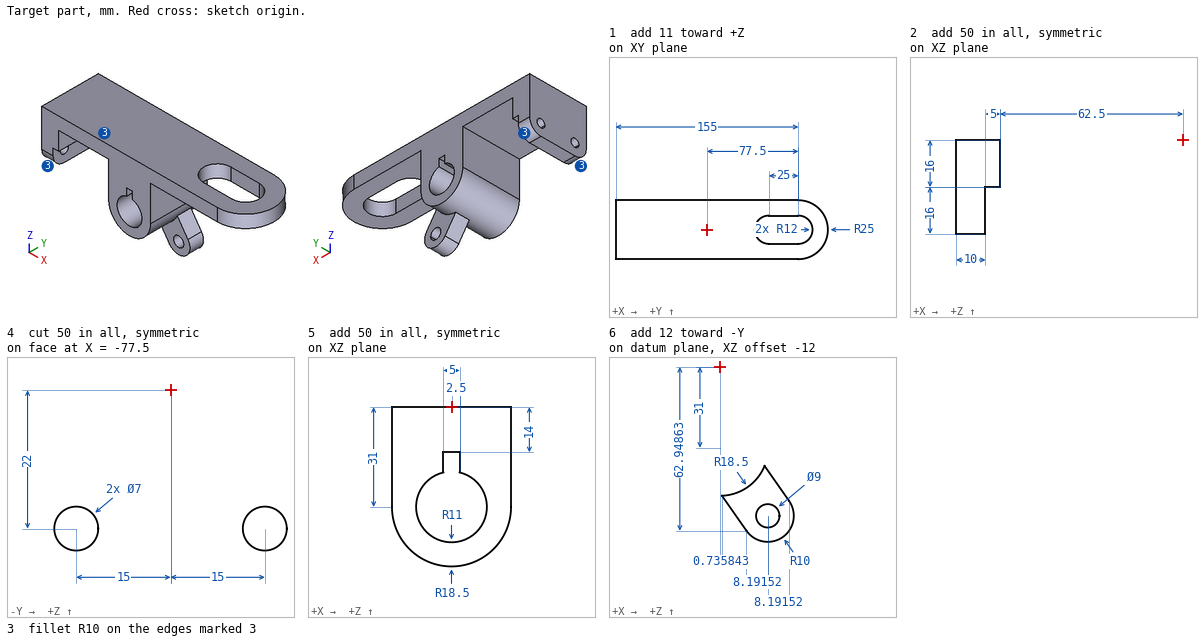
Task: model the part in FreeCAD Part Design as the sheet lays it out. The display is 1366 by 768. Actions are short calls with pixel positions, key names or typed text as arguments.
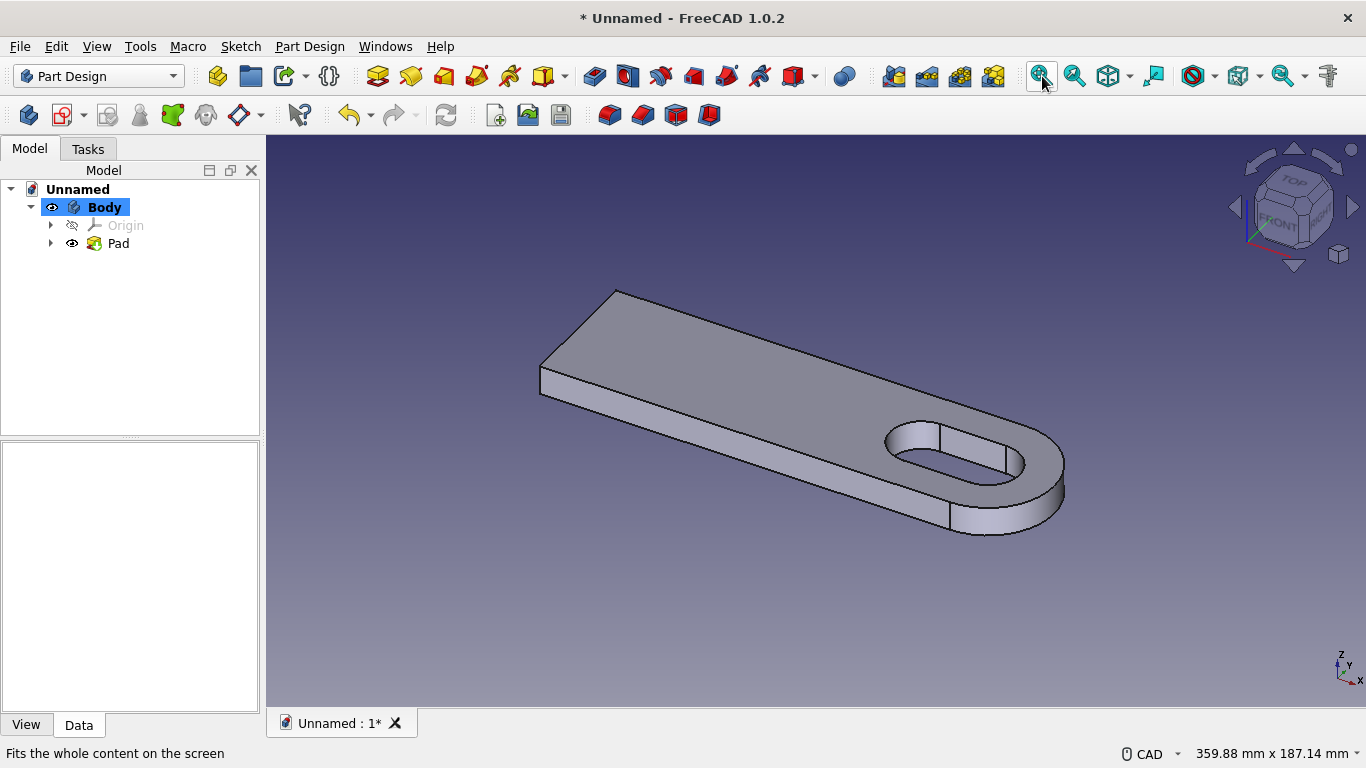
click(62, 116)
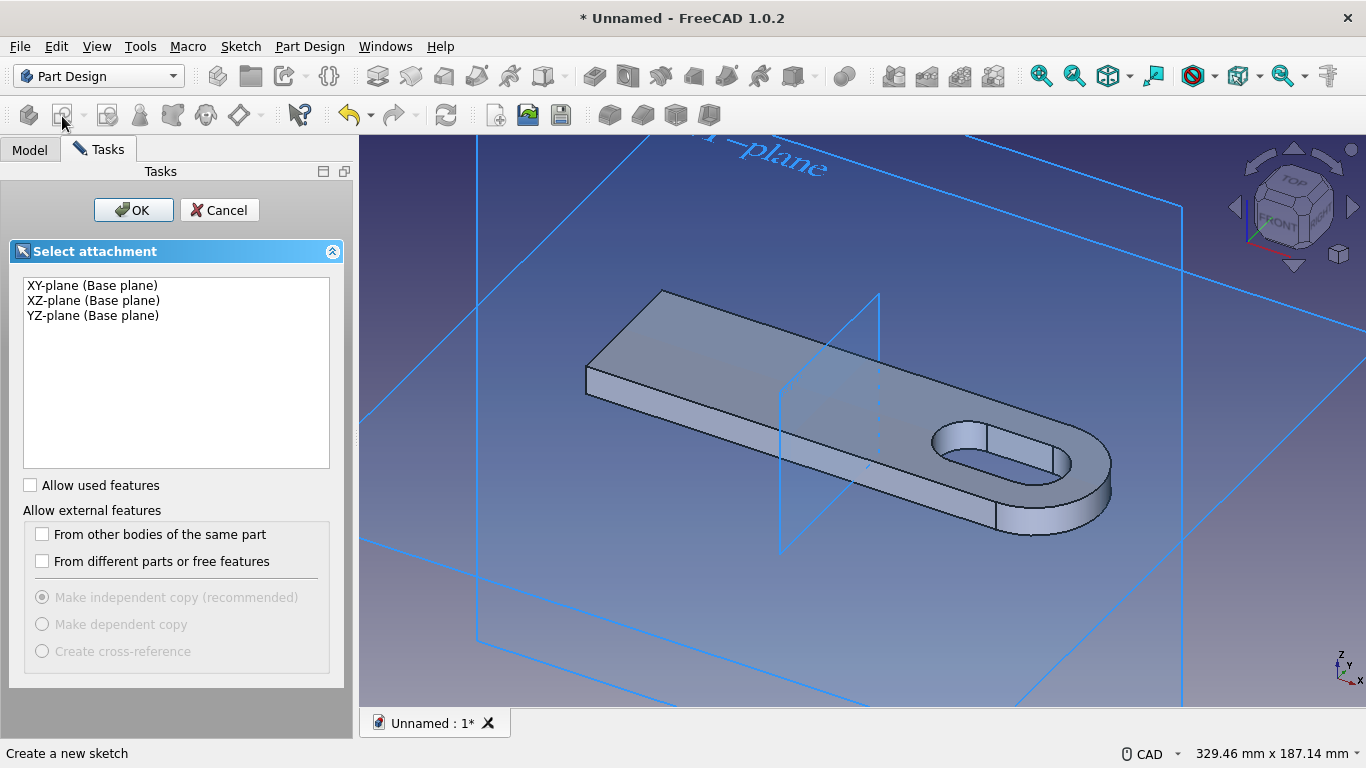
click(84, 300)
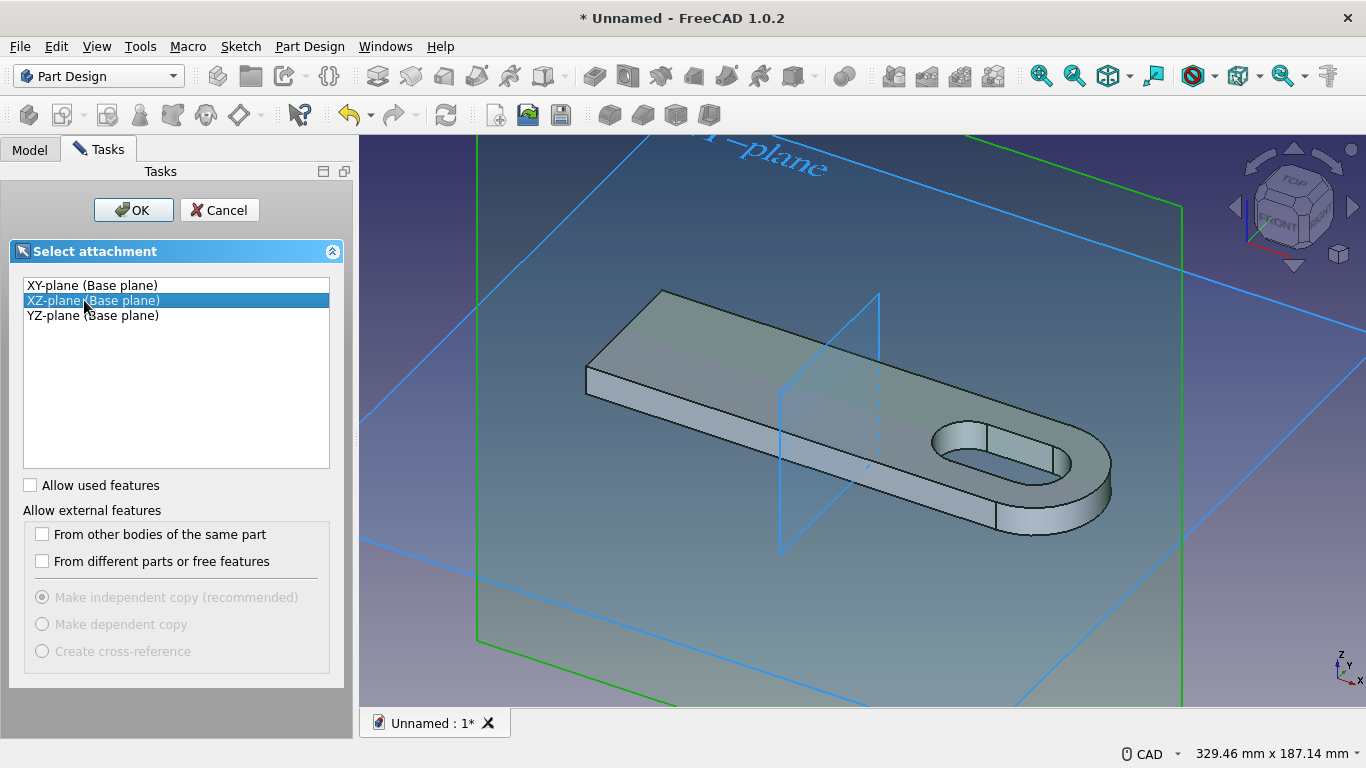
click(134, 210)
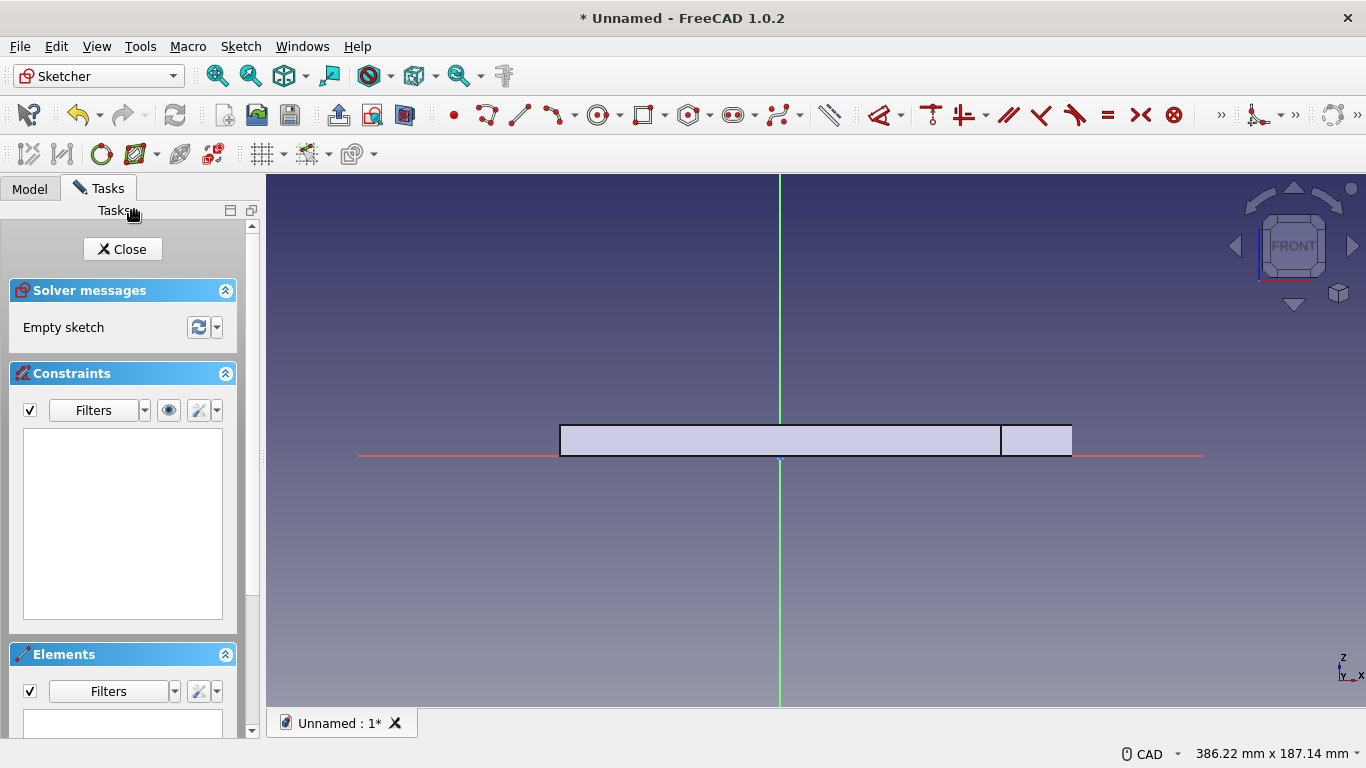
key(q)
key(s)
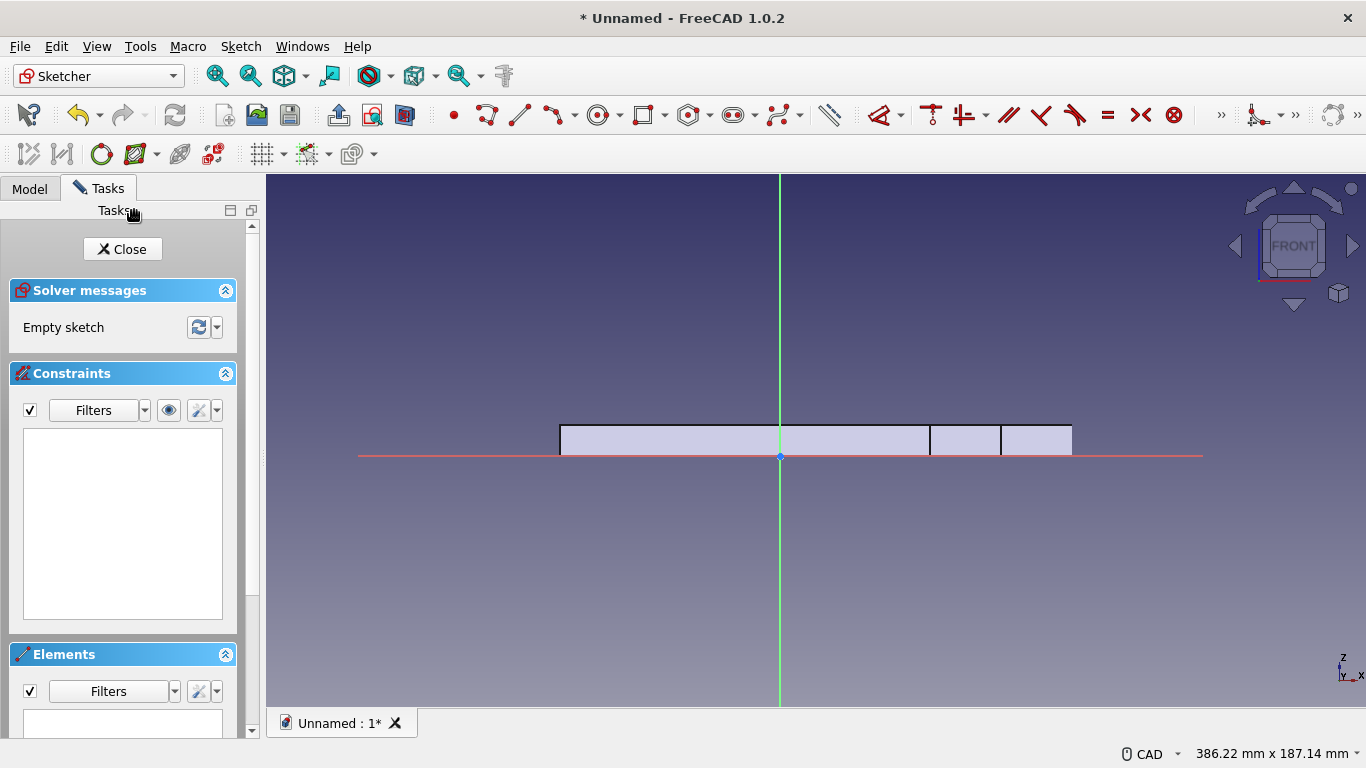
scroll(625, 537, up, 5)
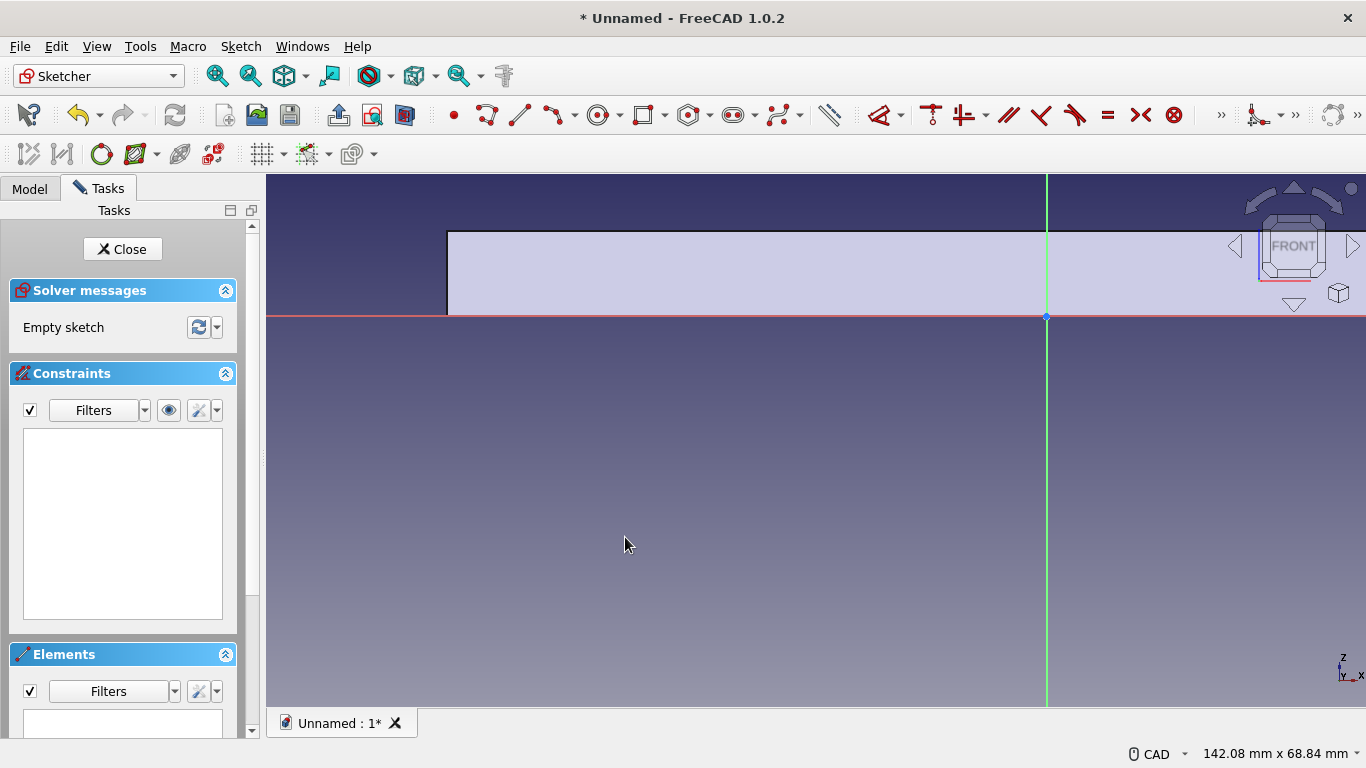
click(487, 116)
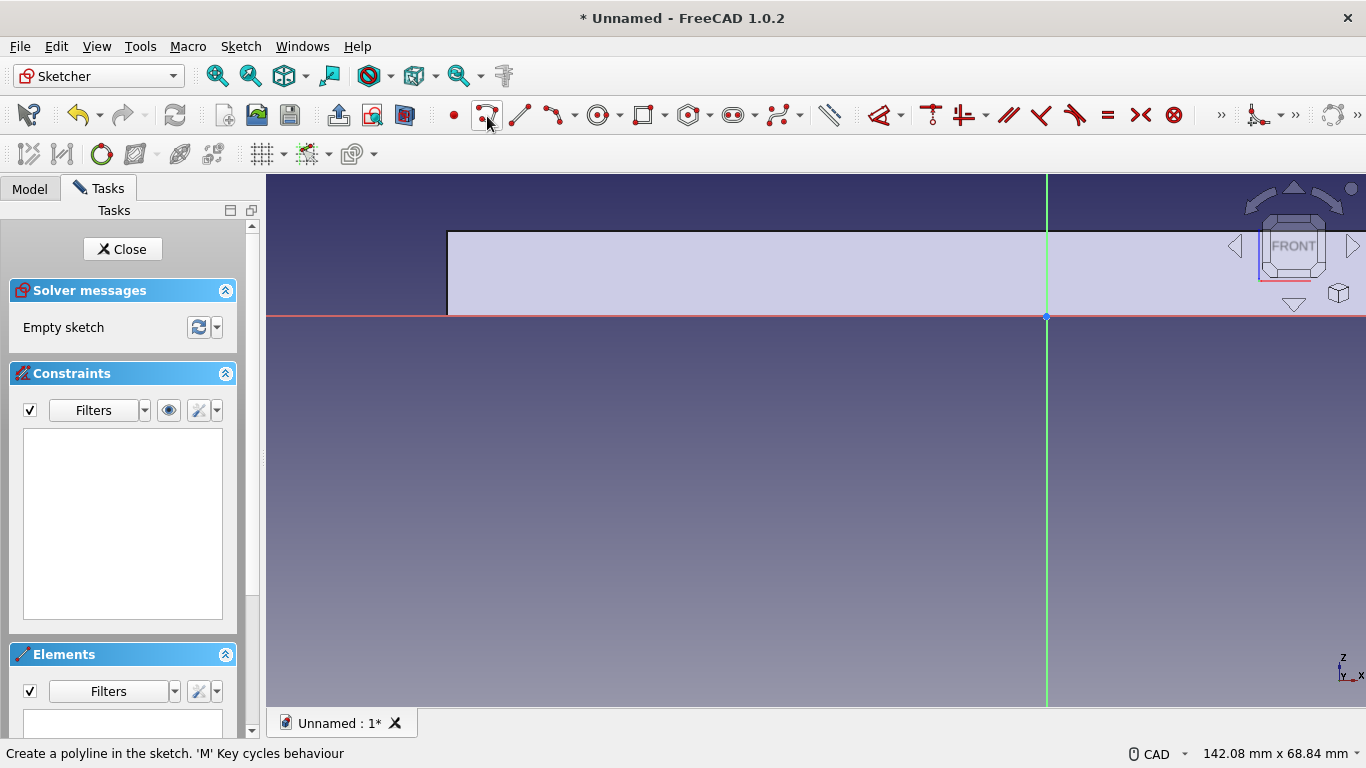
click(563, 316)
click(563, 440)
click(524, 440)
click(524, 564)
click(447, 564)
click(447, 325)
click(563, 316)
key(Escape)
key(Escape)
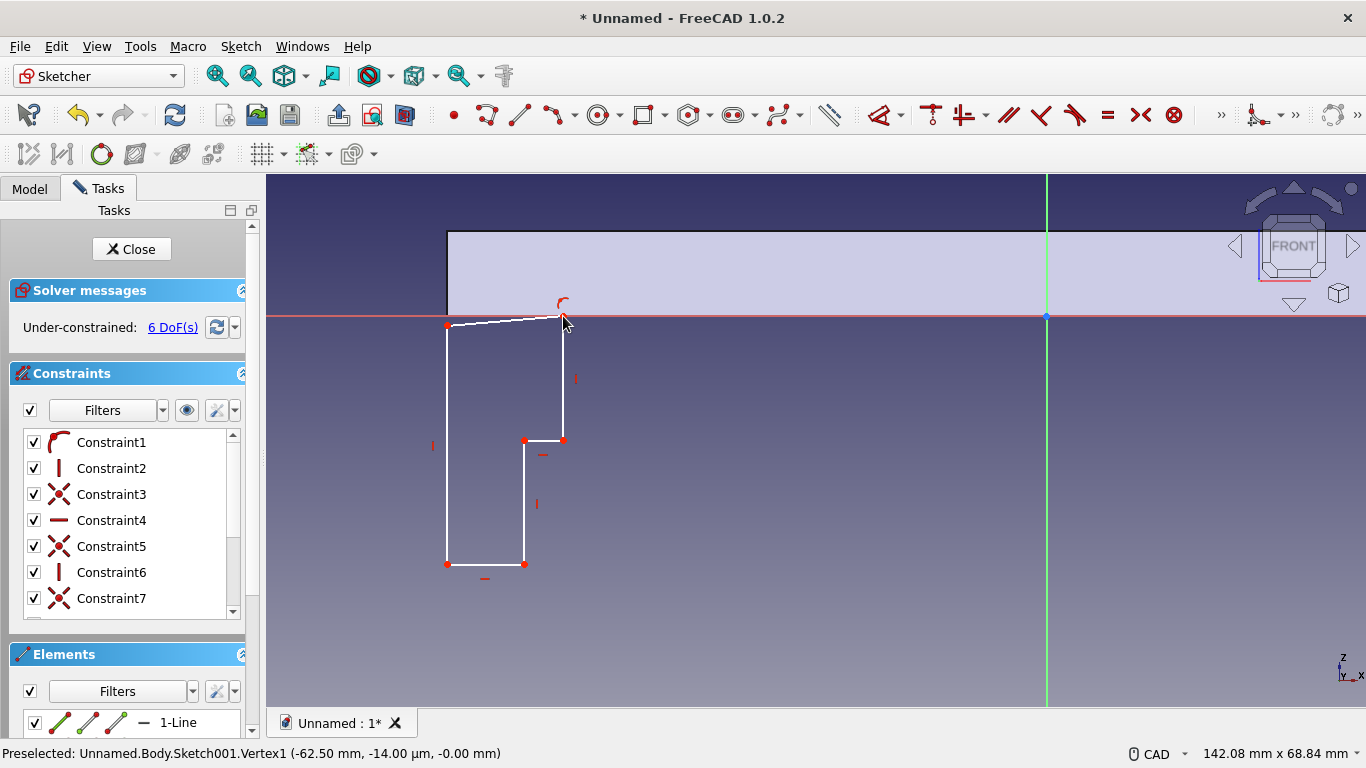
click(528, 319)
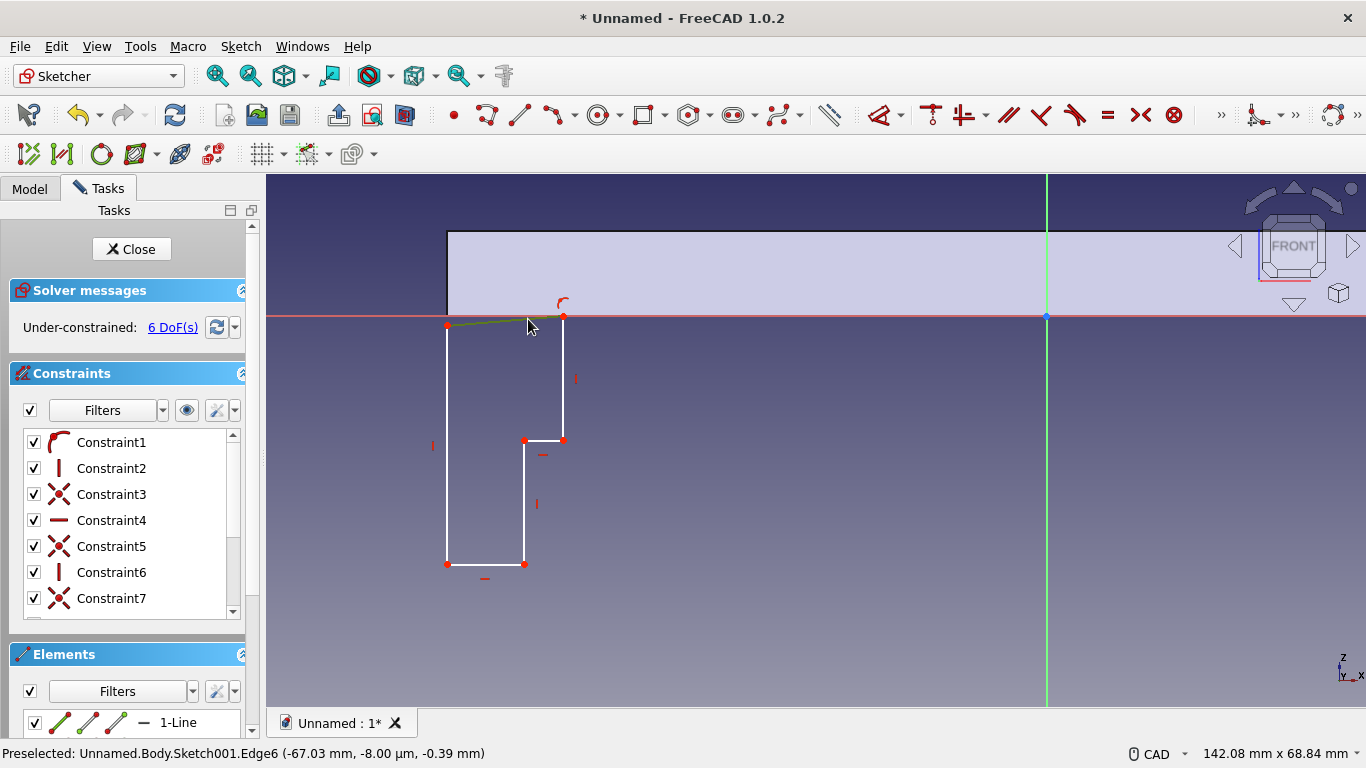
click(986, 116)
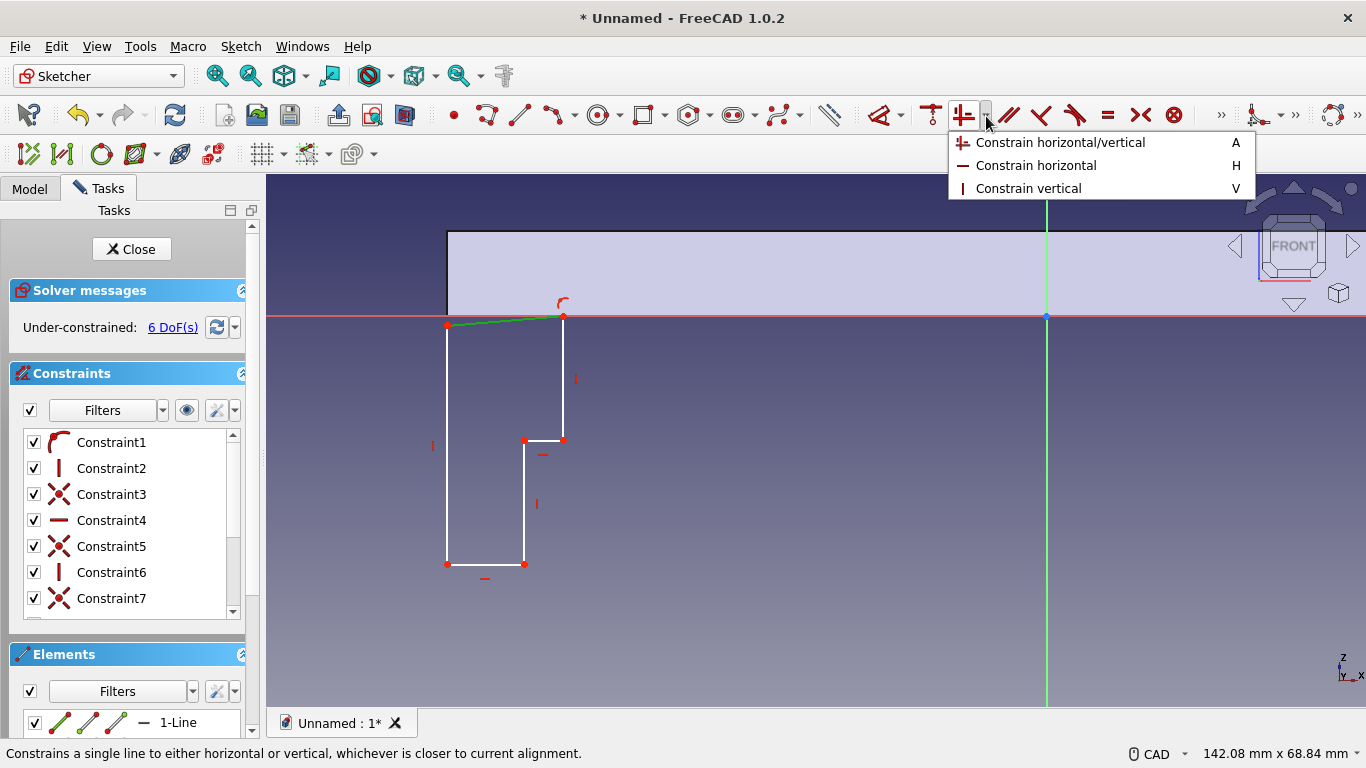
click(1102, 166)